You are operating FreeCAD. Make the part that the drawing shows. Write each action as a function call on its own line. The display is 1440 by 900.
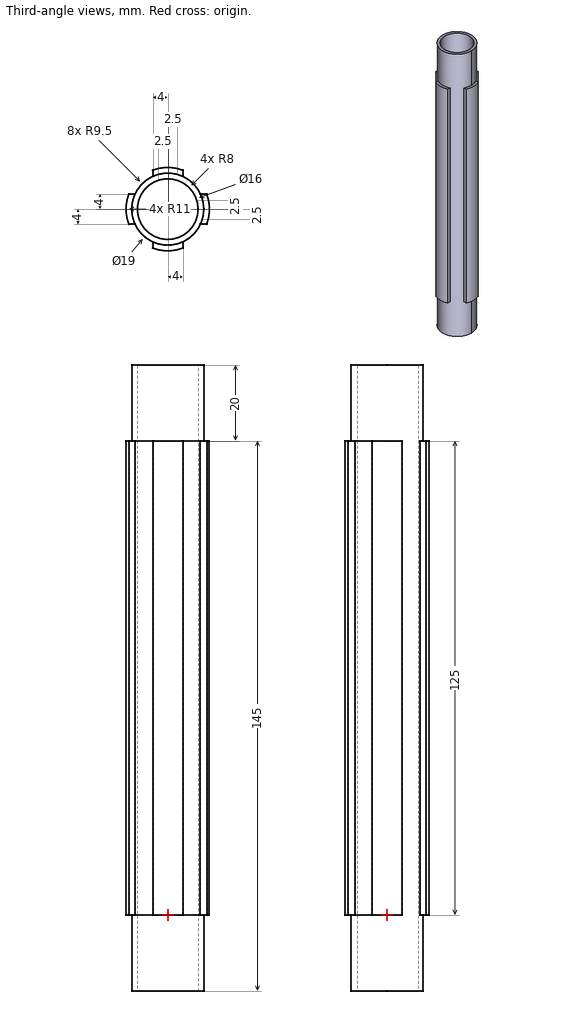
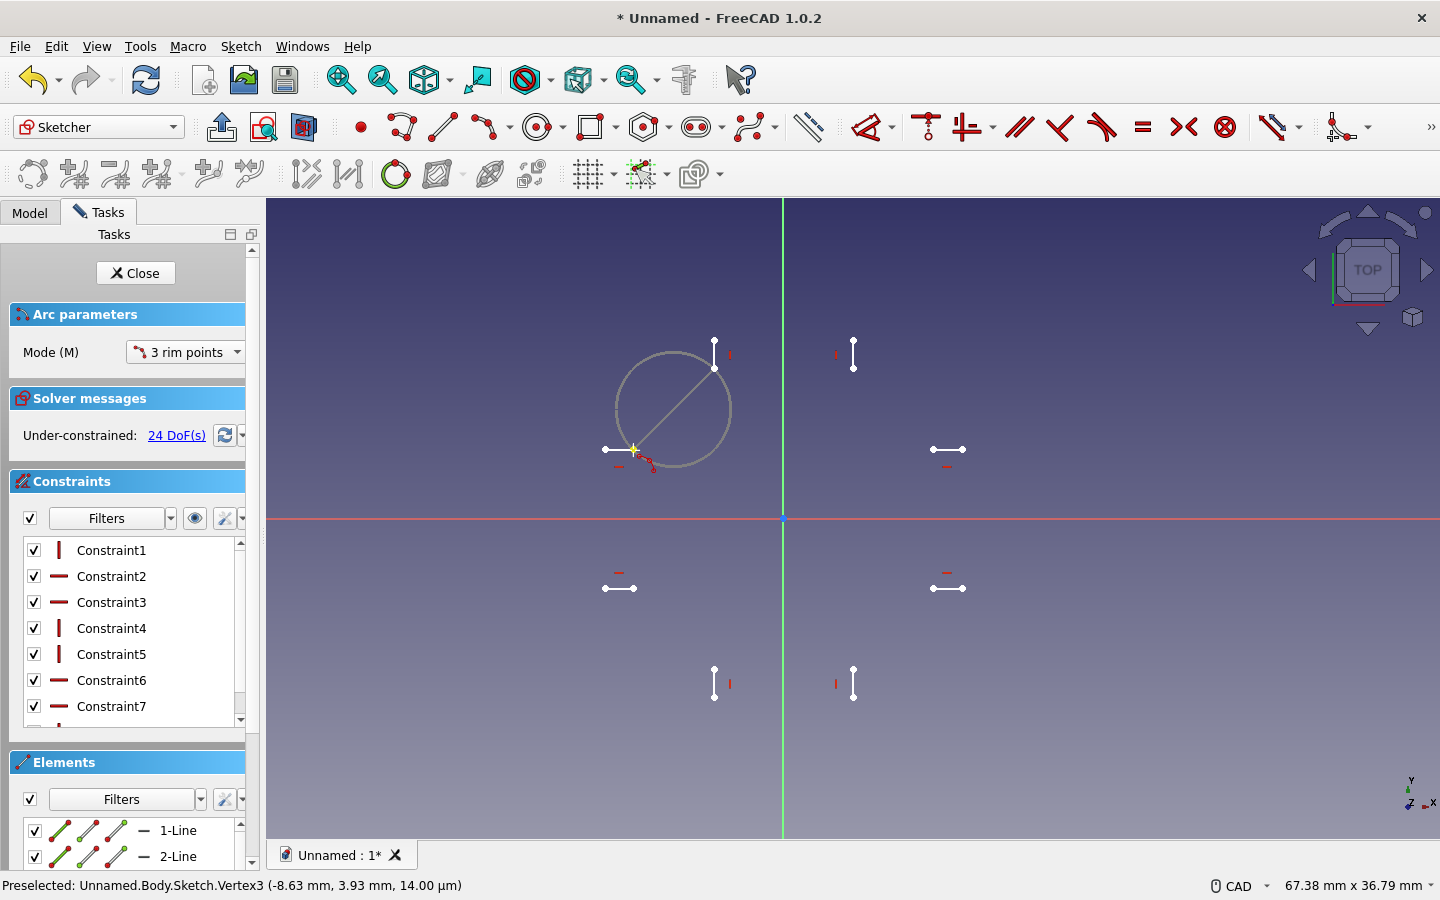
scroll(666, 401, up, 3)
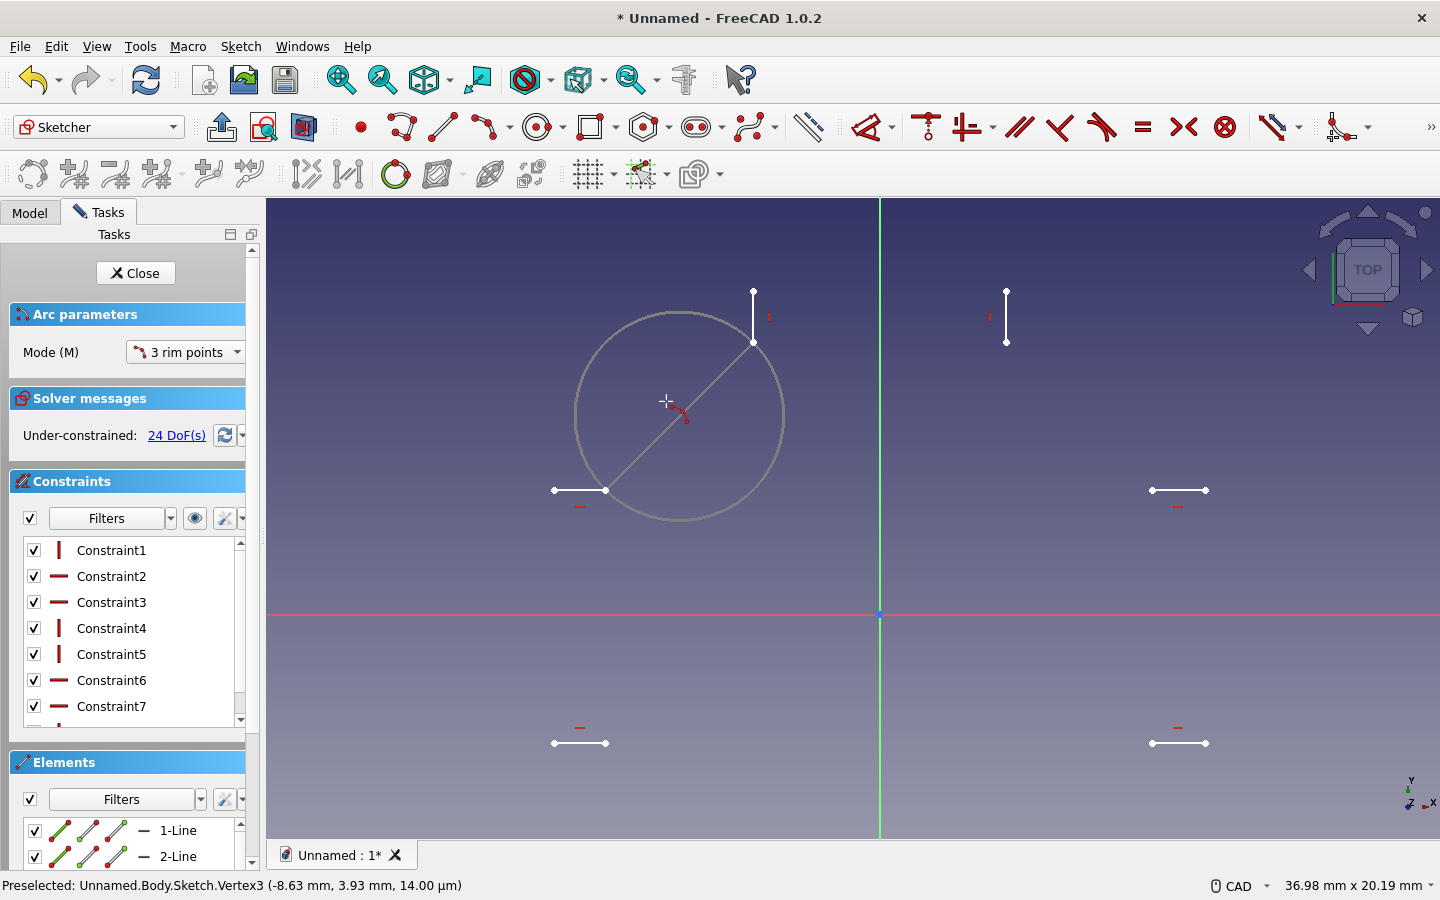
click(666, 402)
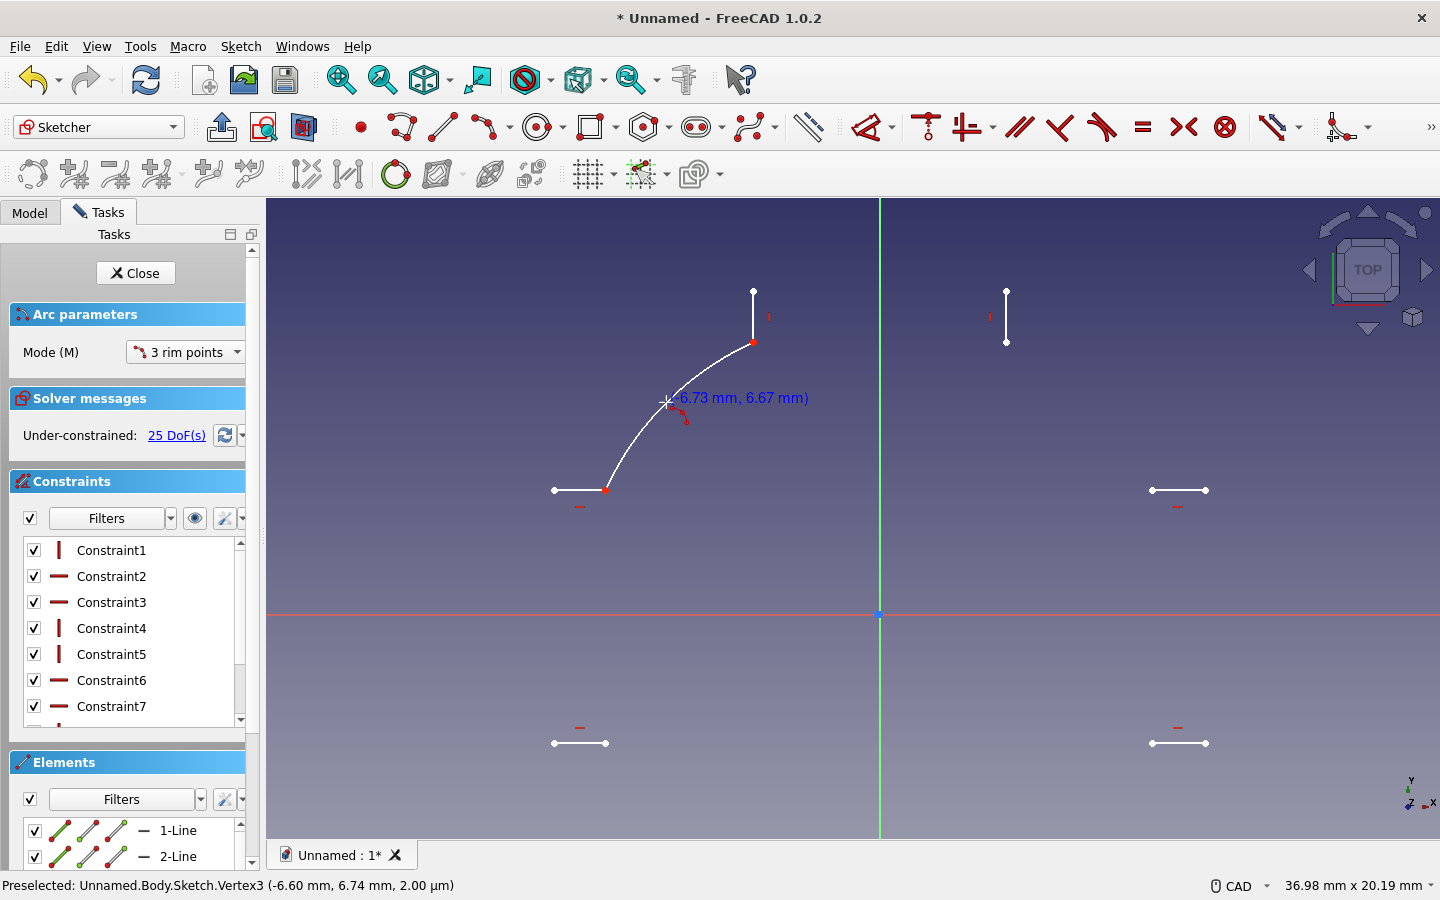
click(555, 490)
click(555, 743)
click(531, 589)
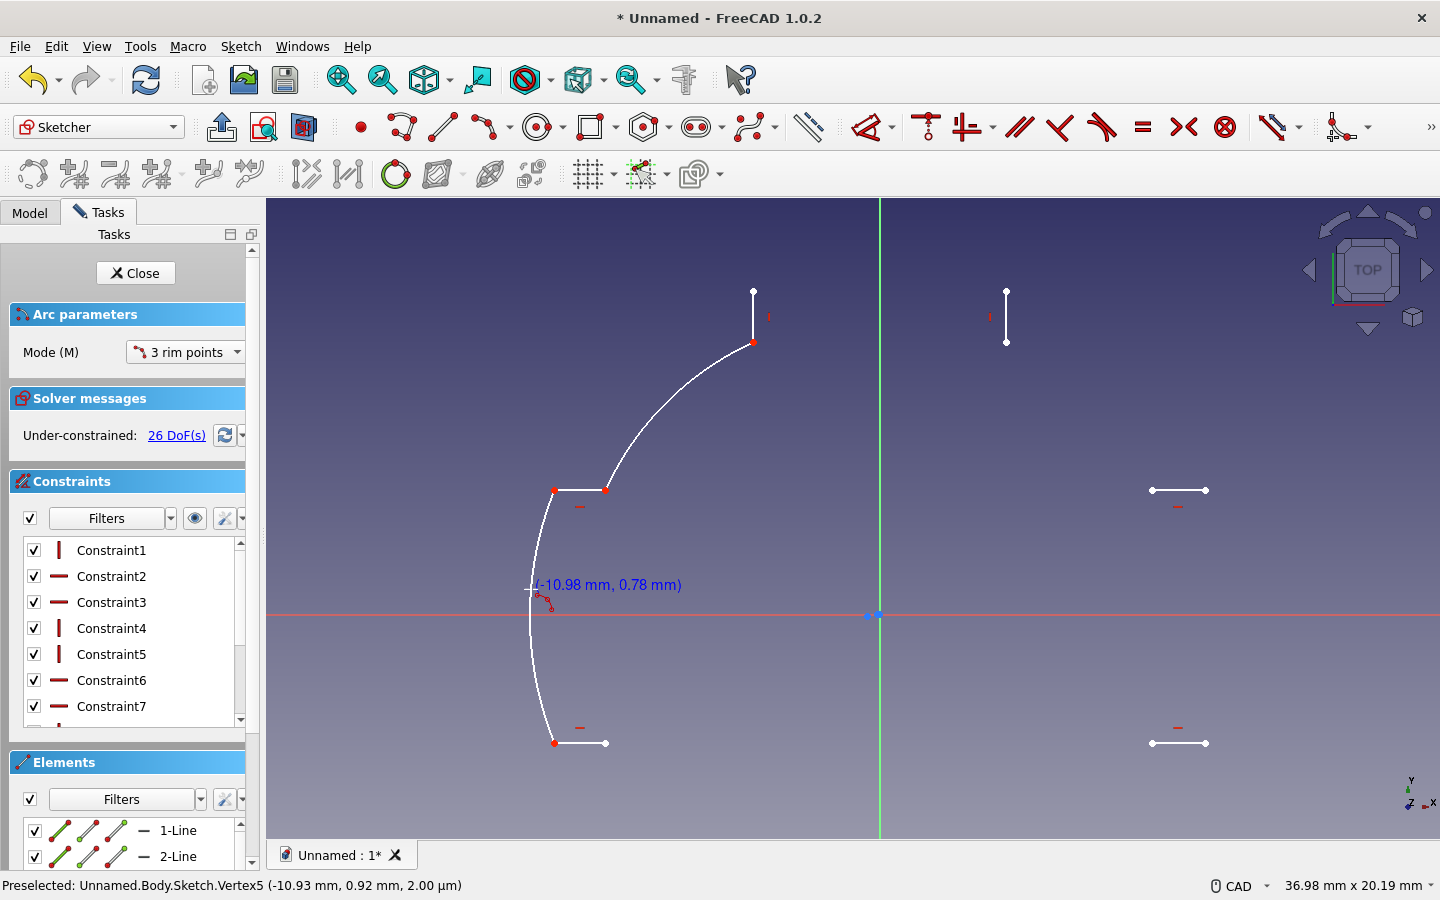
click(606, 743)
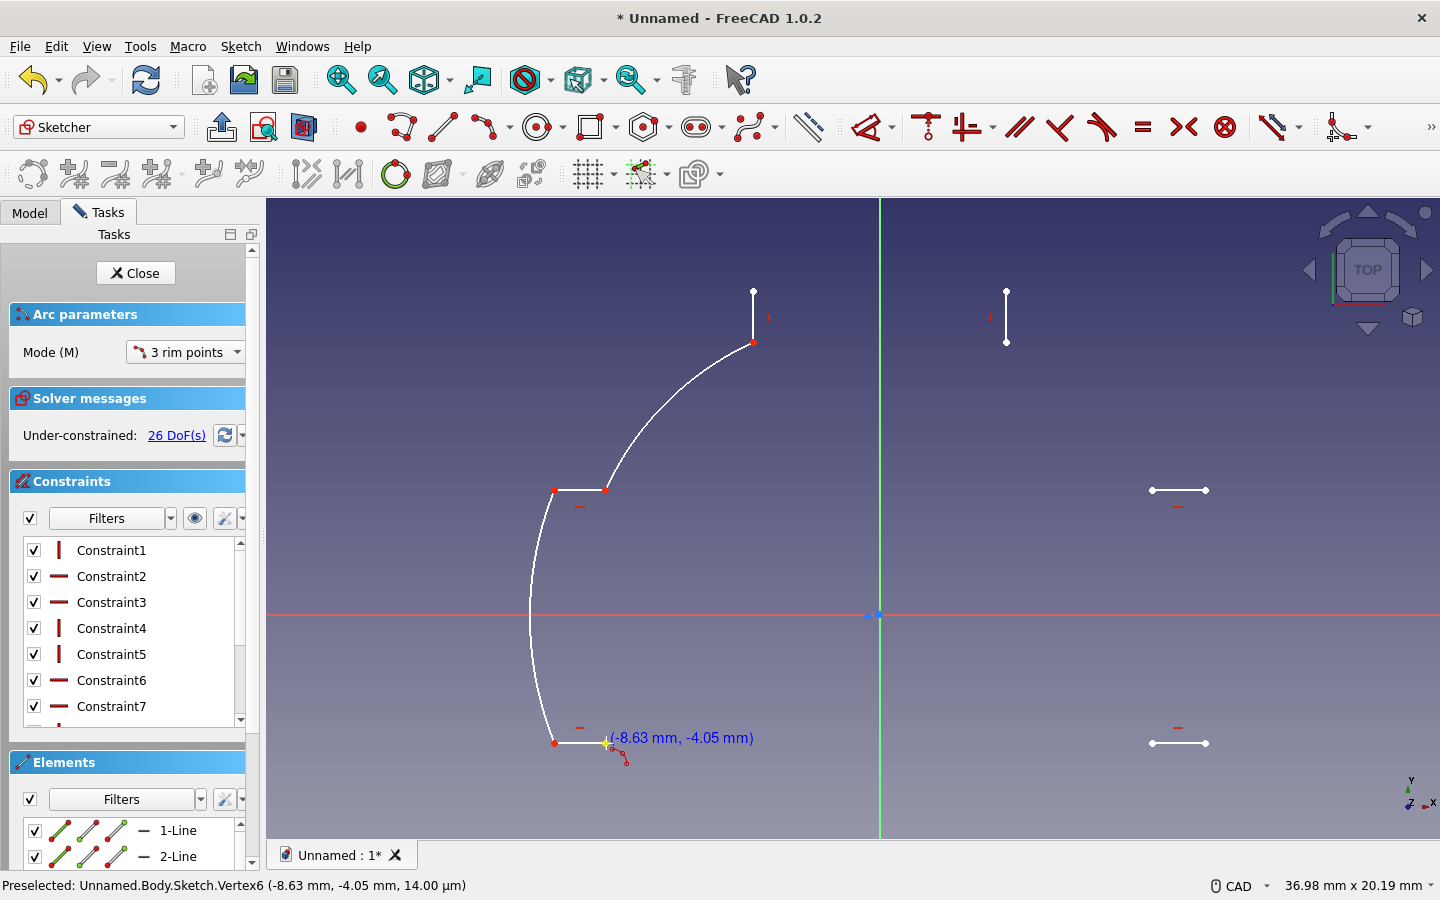
scroll(669, 401, down, 3)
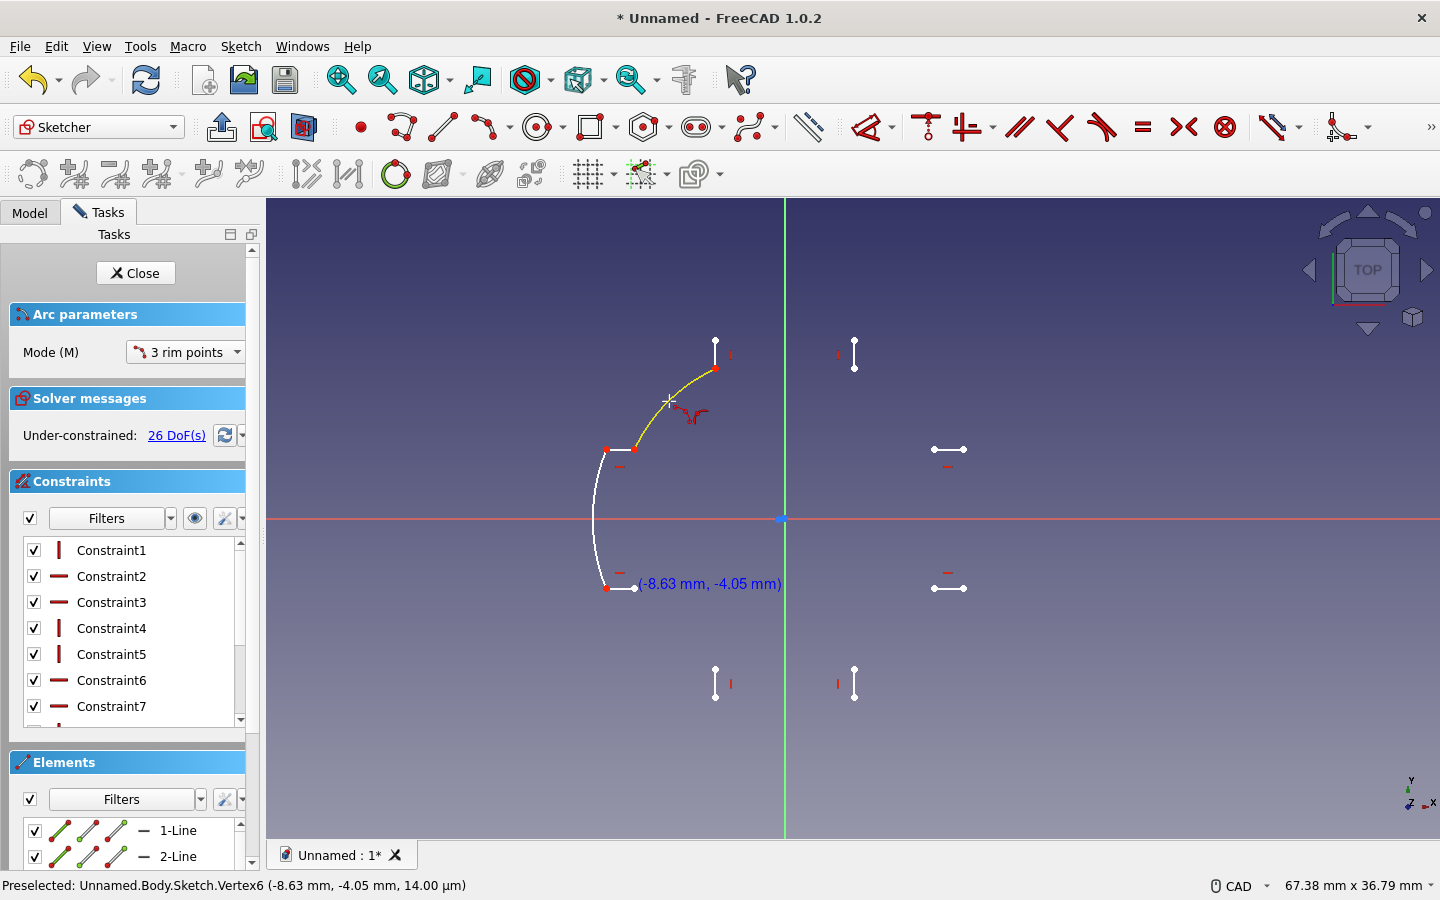
click(715, 670)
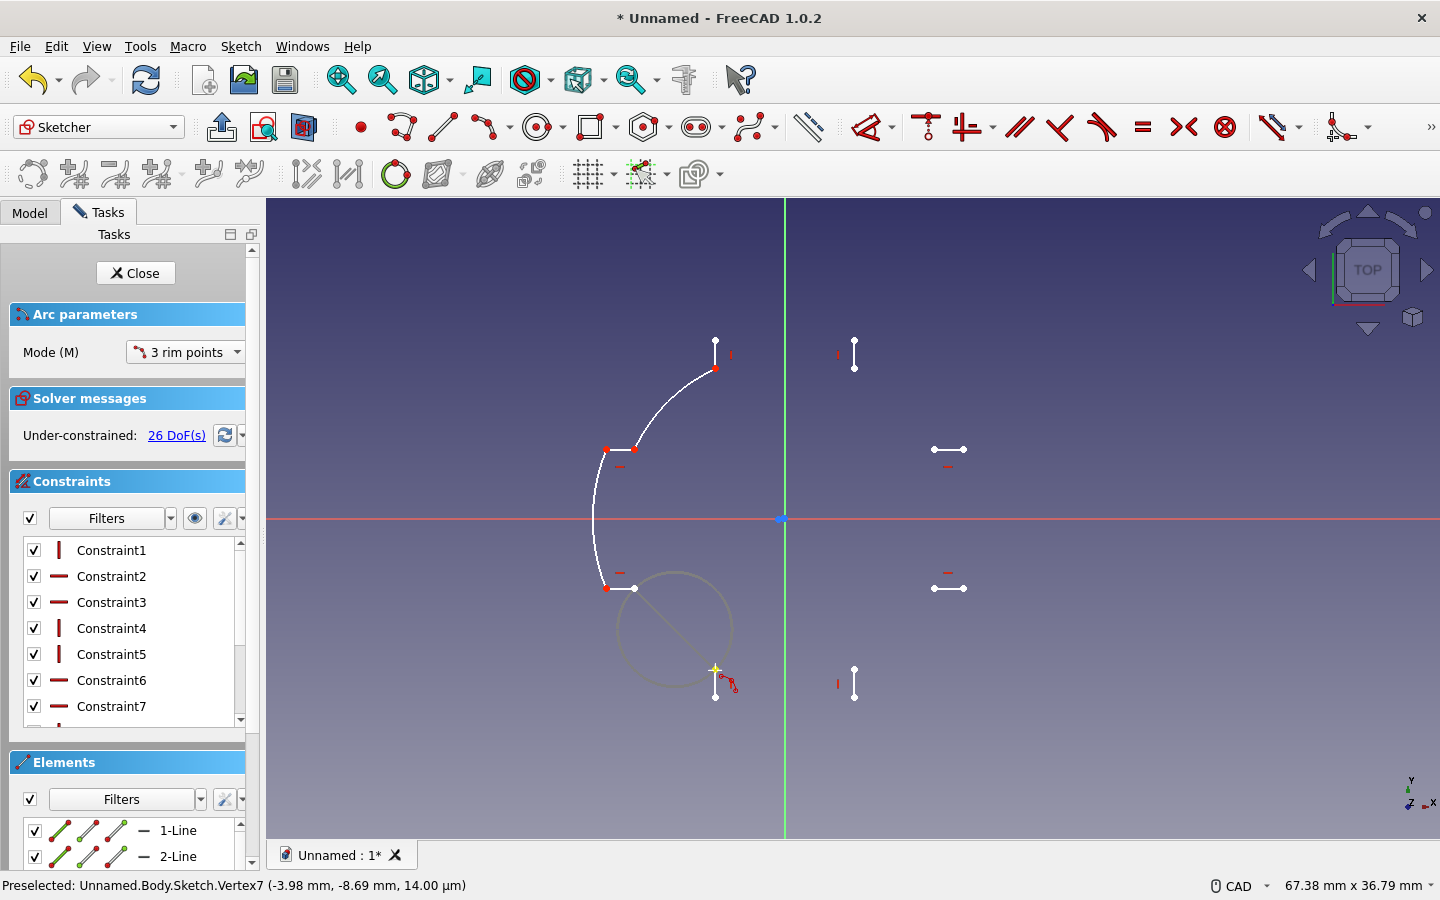
scroll(668, 636, up, 3)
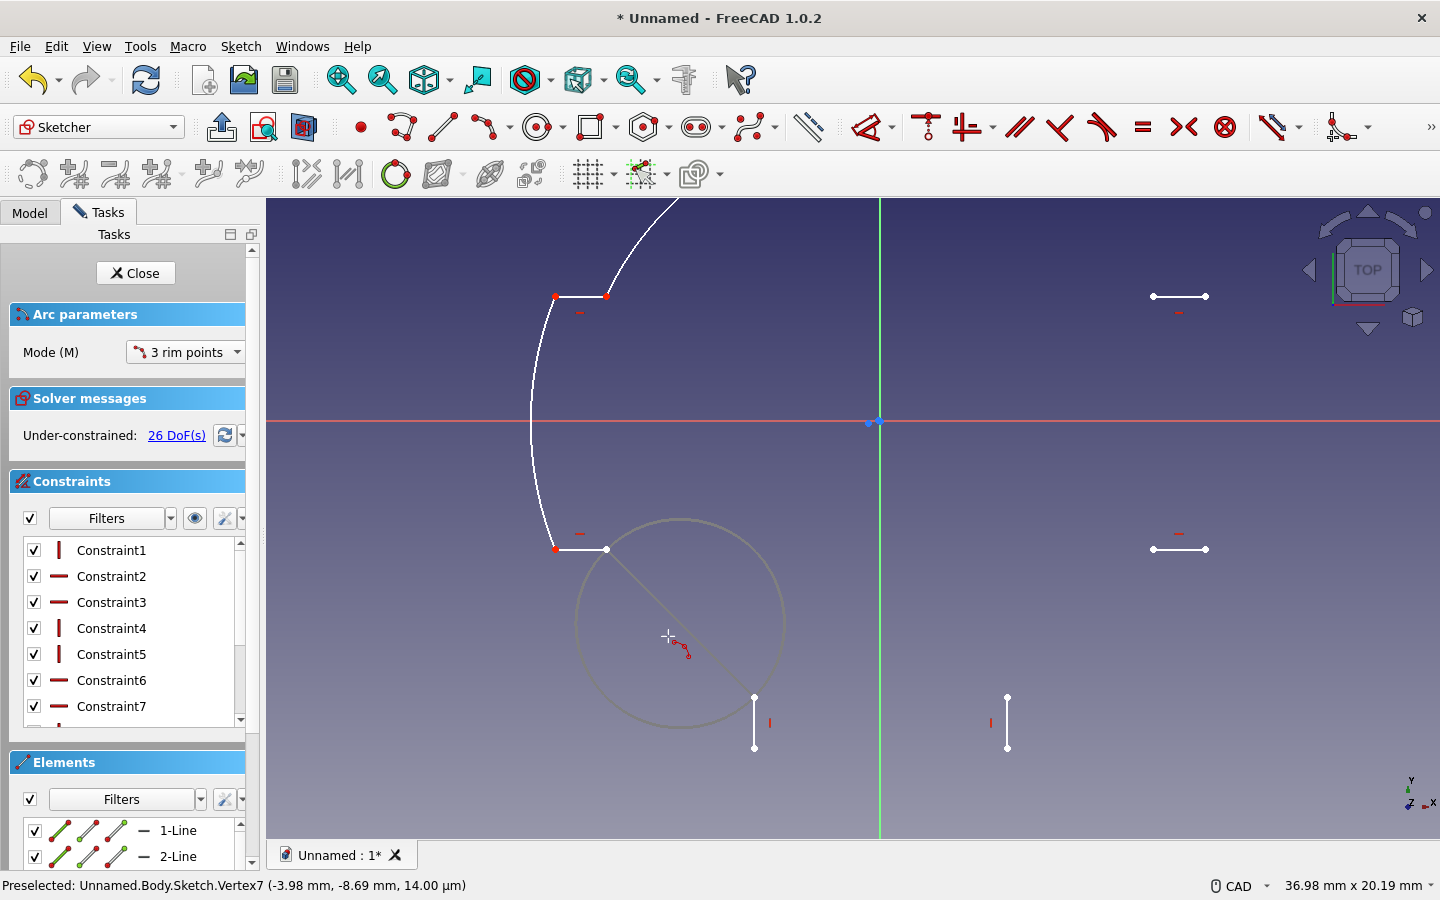
click(667, 635)